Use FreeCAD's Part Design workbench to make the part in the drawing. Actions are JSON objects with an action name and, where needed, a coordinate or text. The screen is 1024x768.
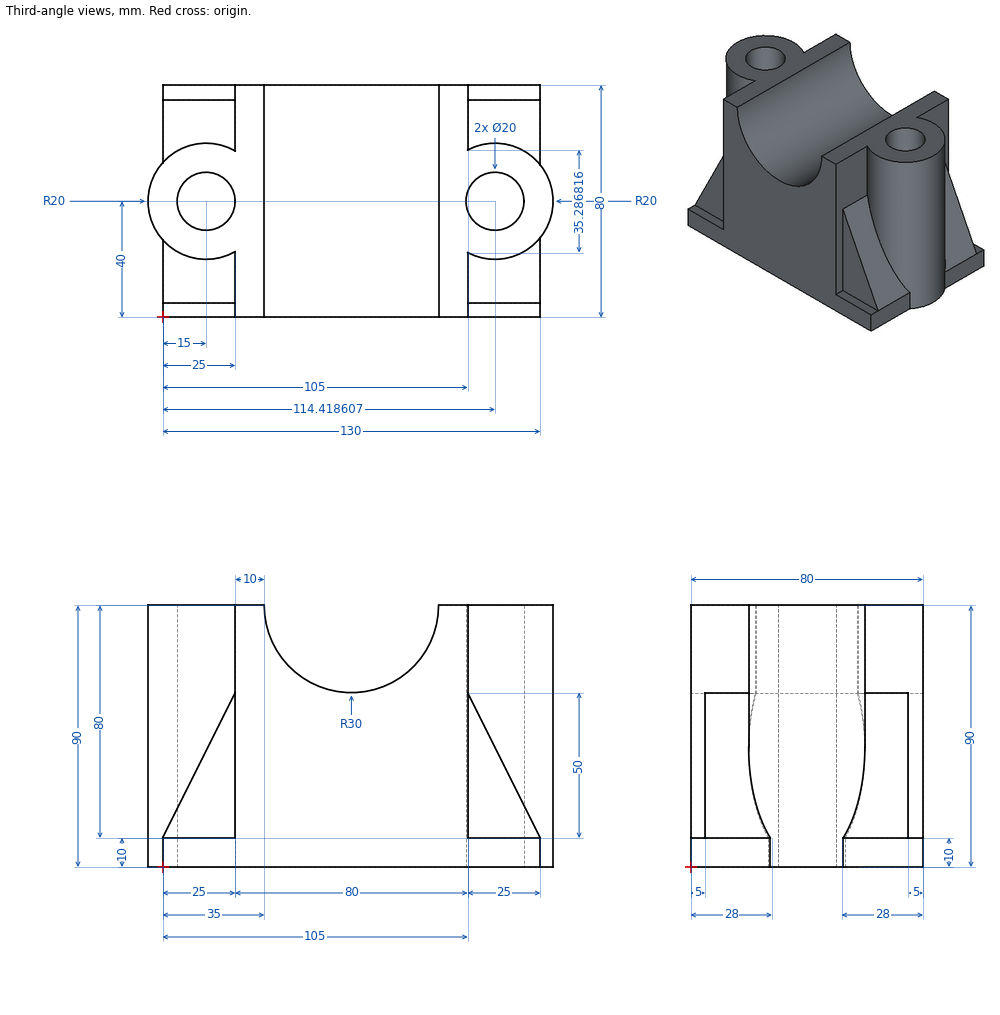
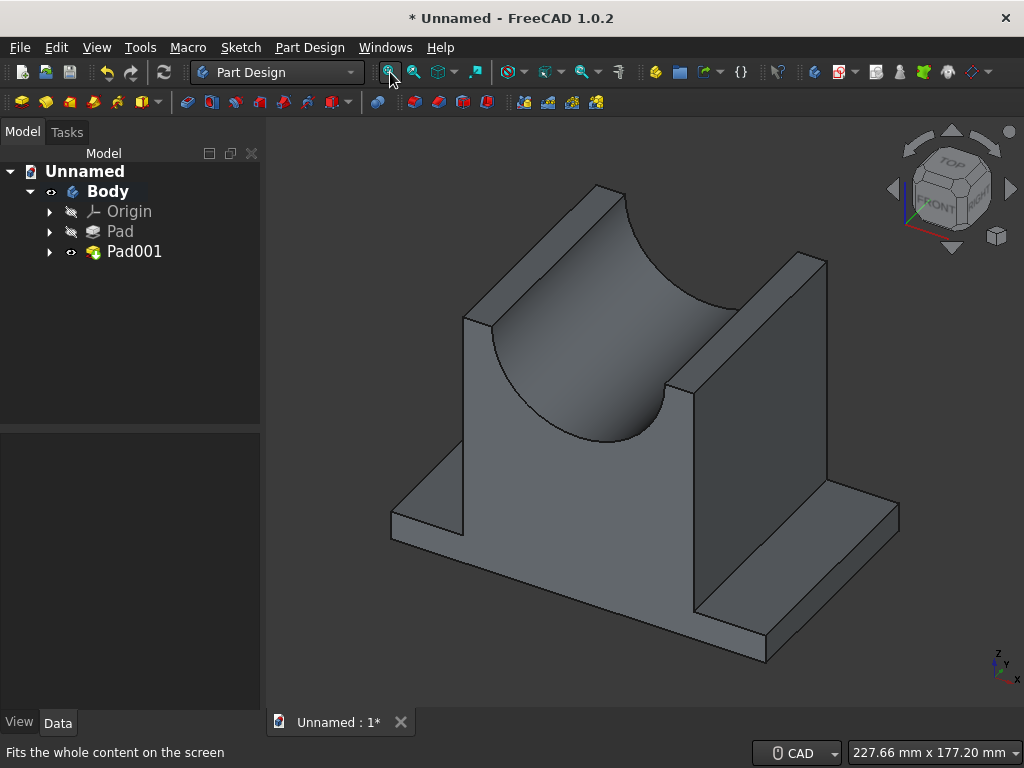
{"action": "left_click", "coordinate": [601, 198]}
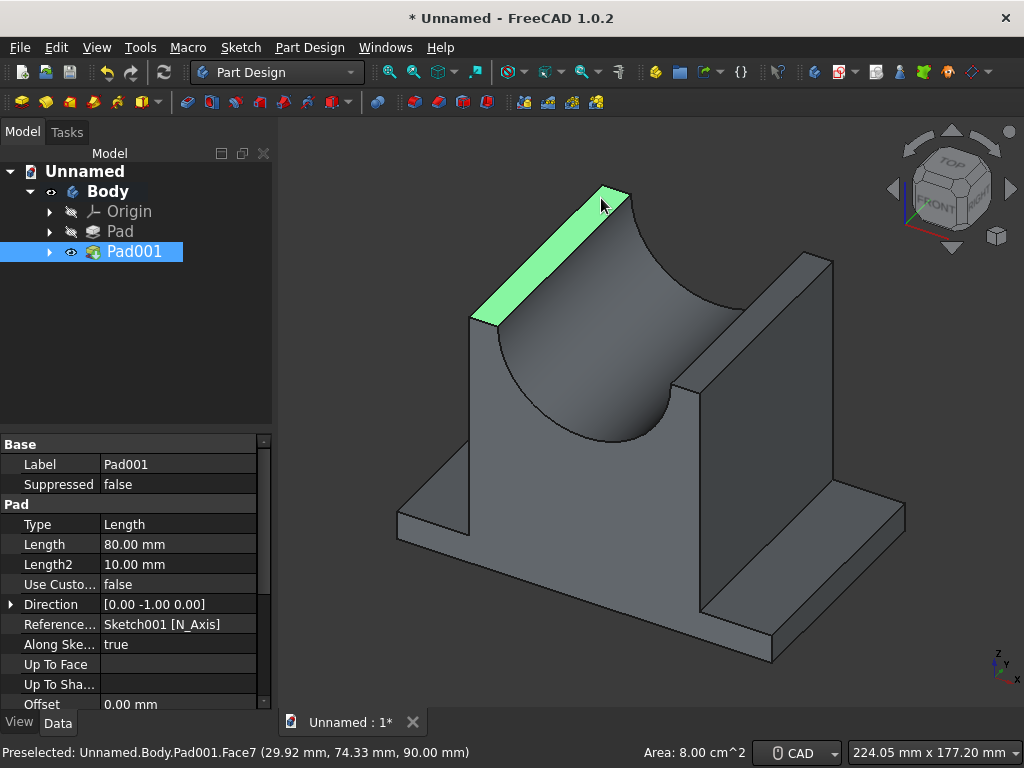
{"action": "left_click", "coordinate": [840, 72]}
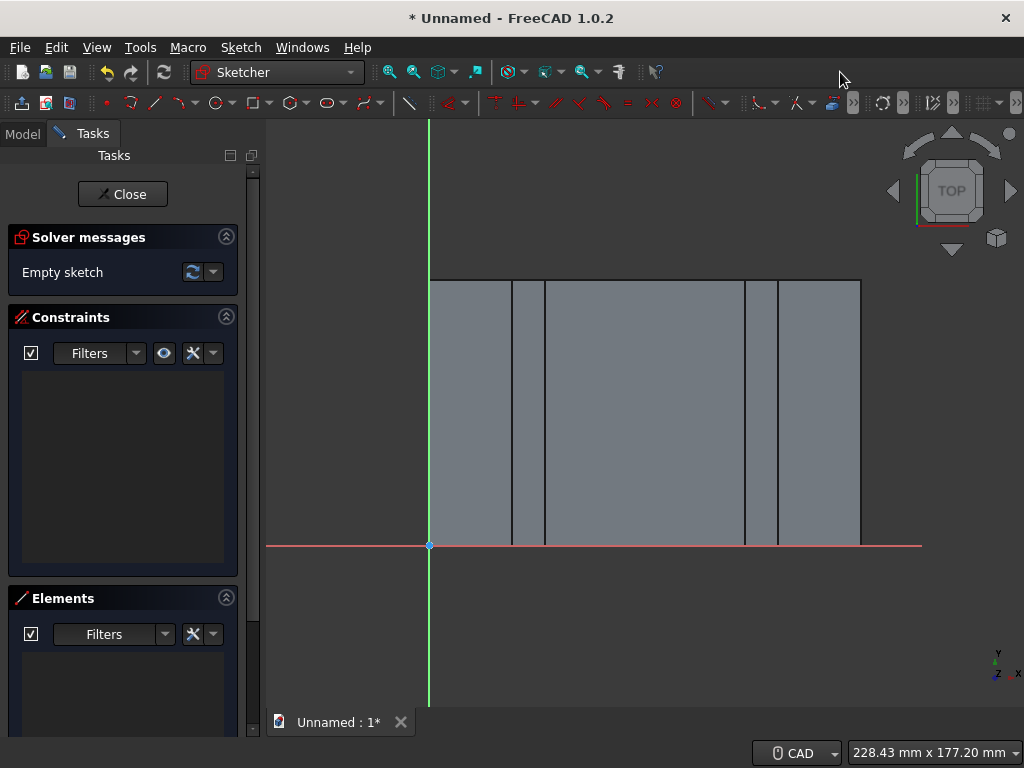
{"action": "scroll", "coordinate": [576, 413], "scroll_direction": "down", "scroll_amount": 5}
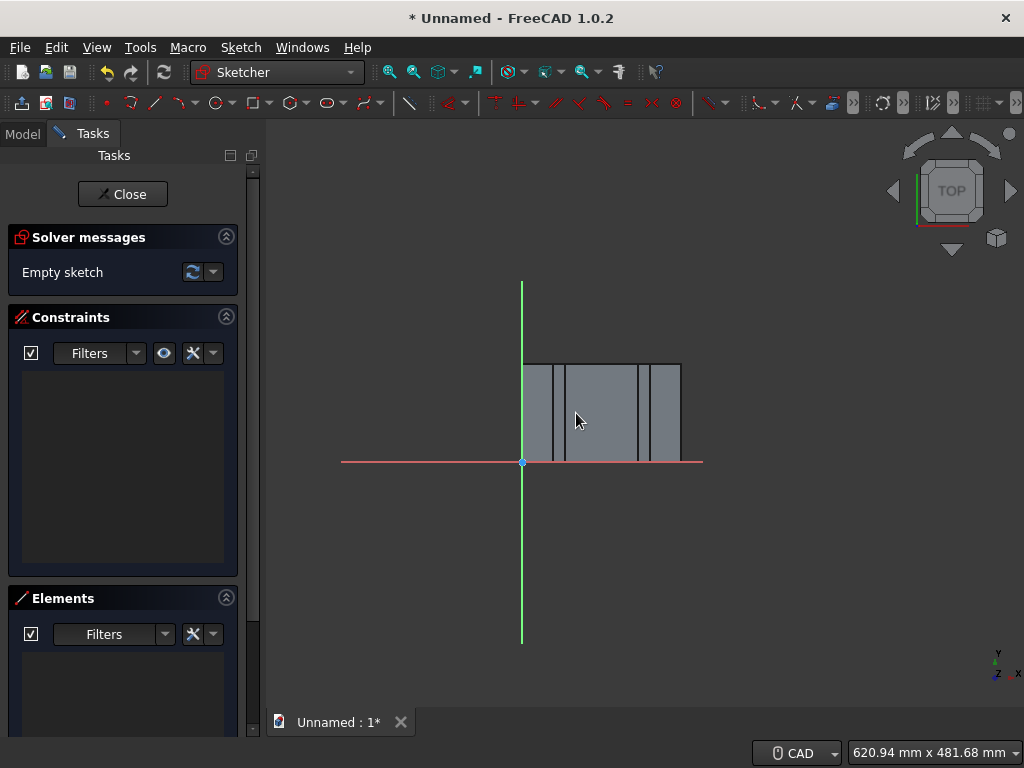
{"action": "scroll", "coordinate": [680, 413], "scroll_direction": "up", "scroll_amount": 11}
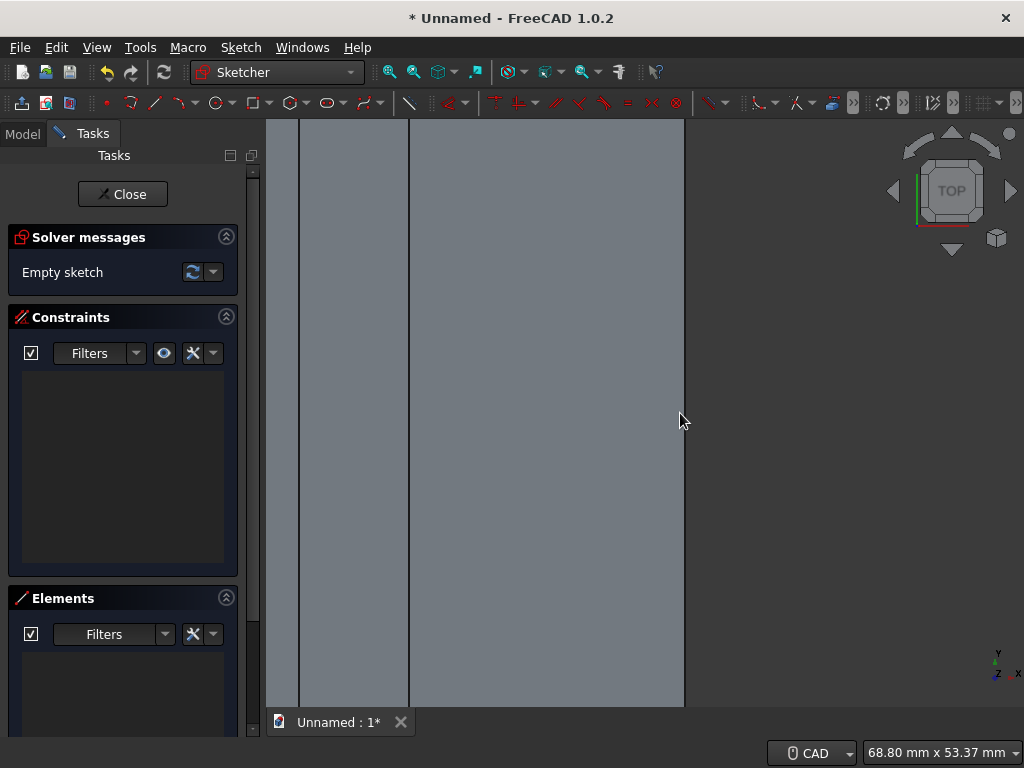
{"action": "left_click", "coordinate": [156, 104]}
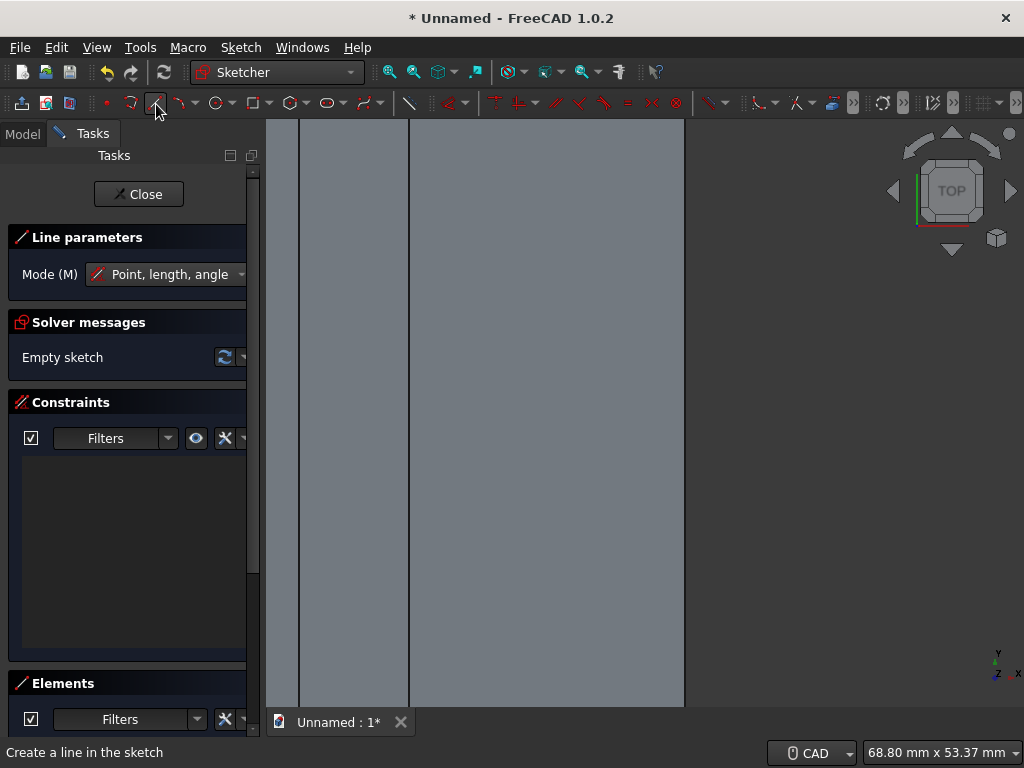
{"action": "left_click", "coordinate": [409, 217]}
{"action": "left_click", "coordinate": [409, 606]}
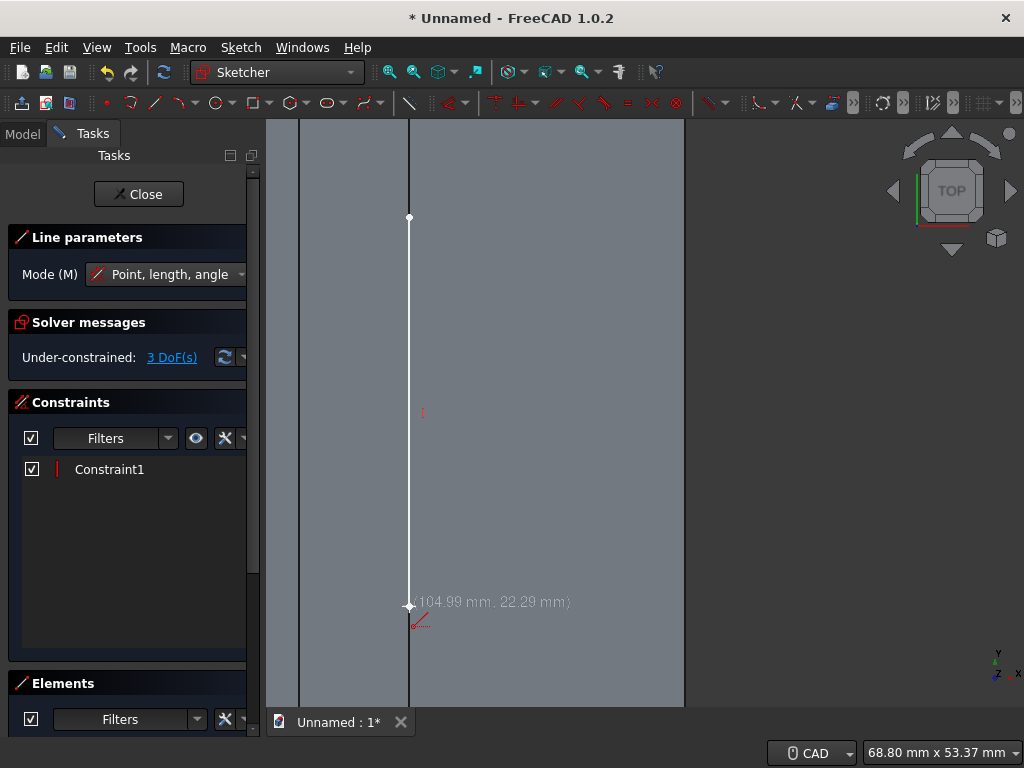
{"action": "left_click", "coordinate": [180, 104]}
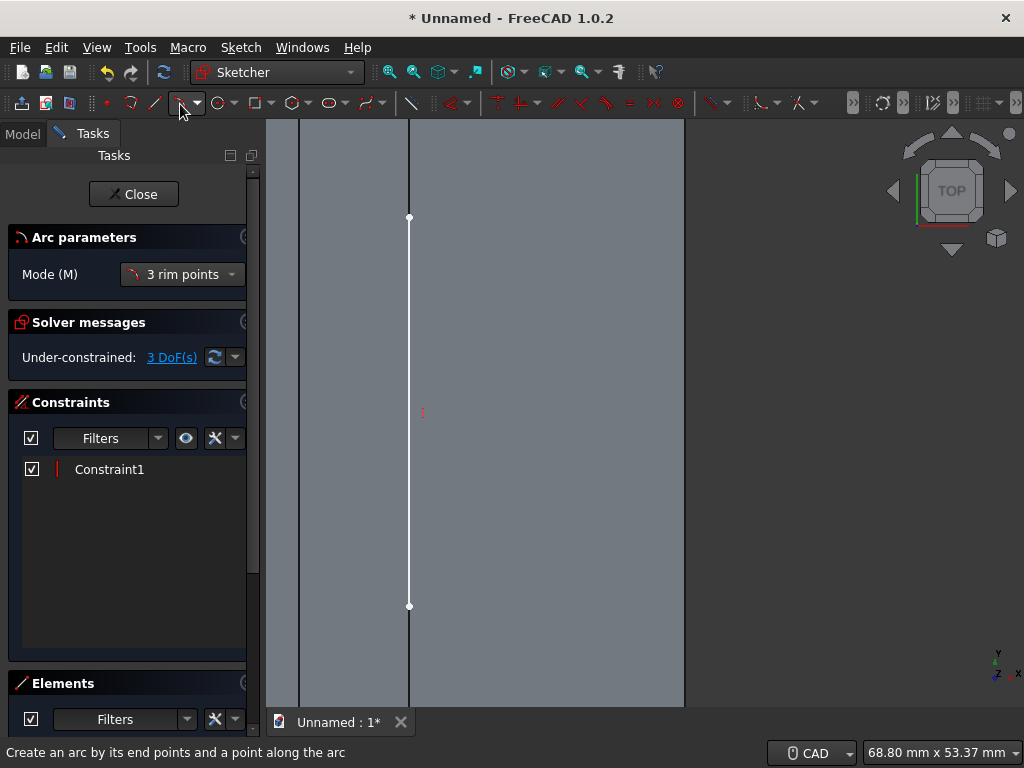
{"action": "left_click", "coordinate": [409, 607]}
{"action": "left_click", "coordinate": [409, 218]}
{"action": "left_click", "coordinate": [733, 412]}
{"action": "key", "text": "Escape"}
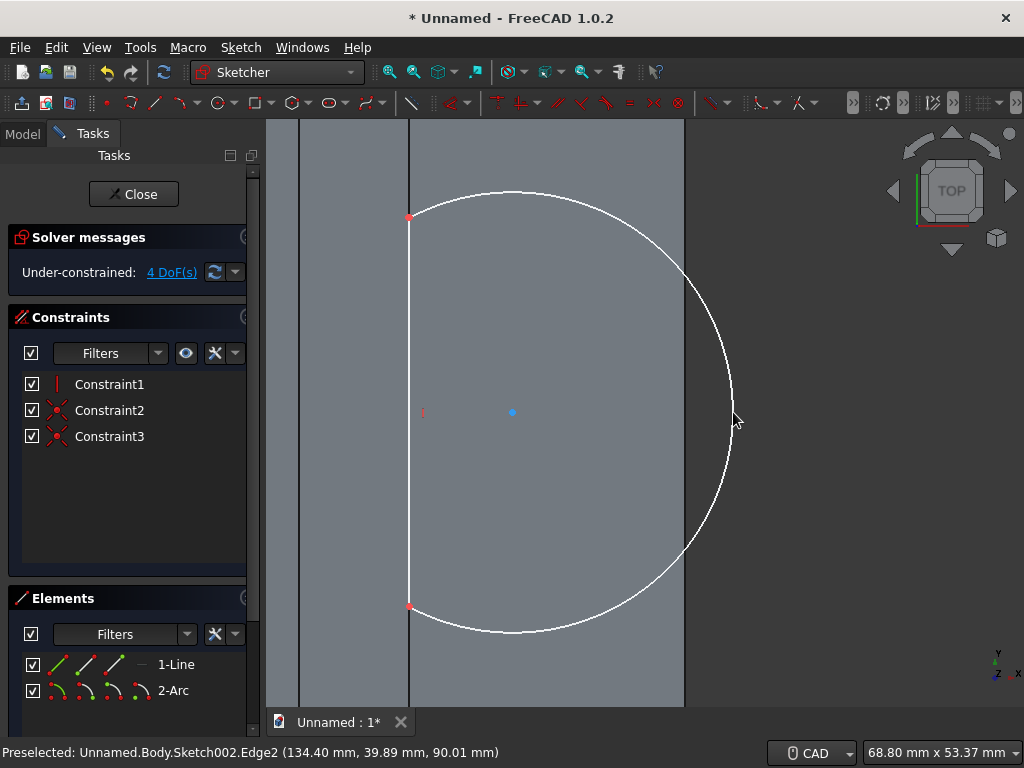
{"action": "left_click", "coordinate": [450, 104]}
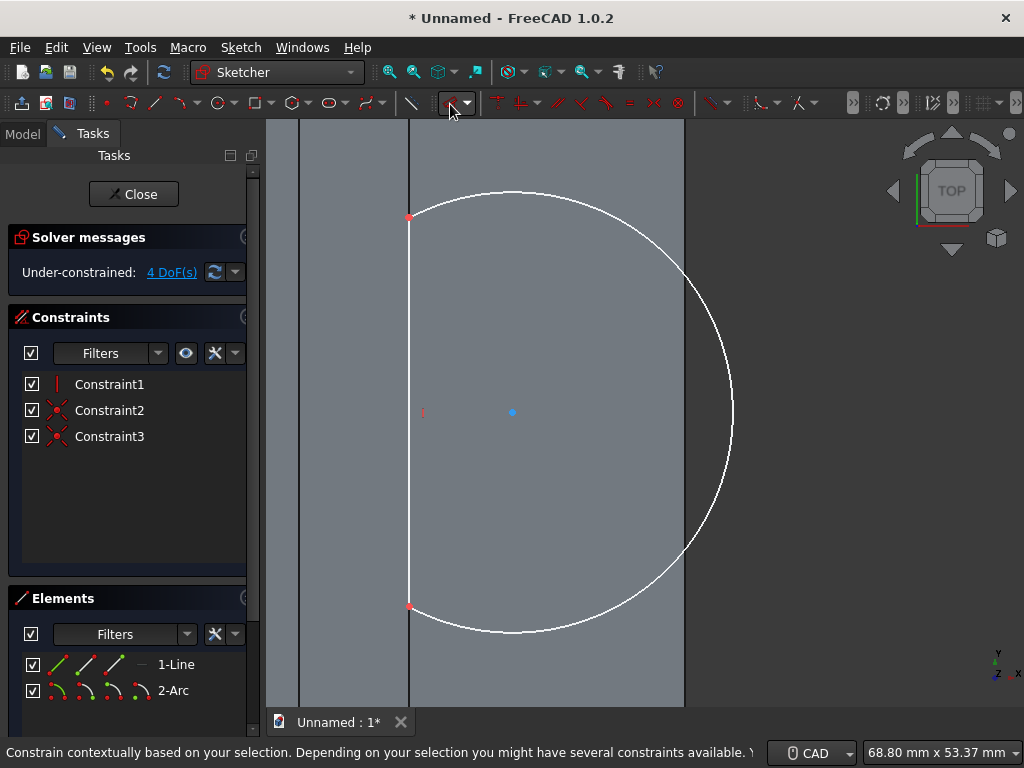
{"action": "left_click", "coordinate": [662, 574]}
{"action": "left_click", "coordinate": [684, 597]}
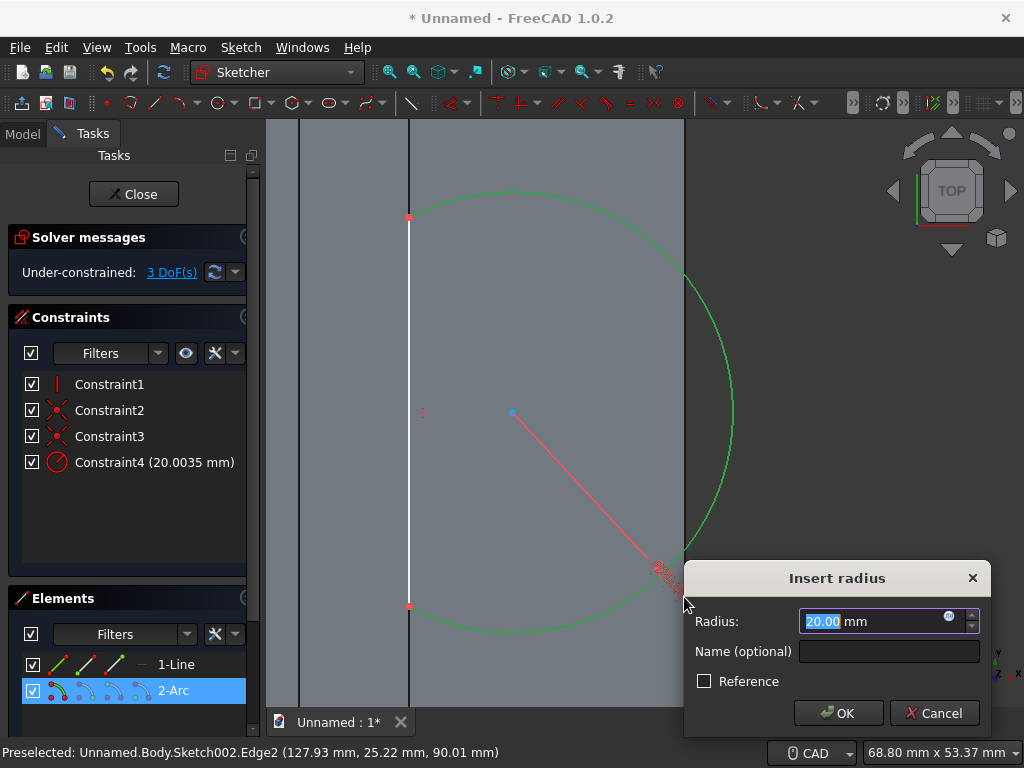
{"action": "type", "text": "20"}
{"action": "key", "text": "Return"}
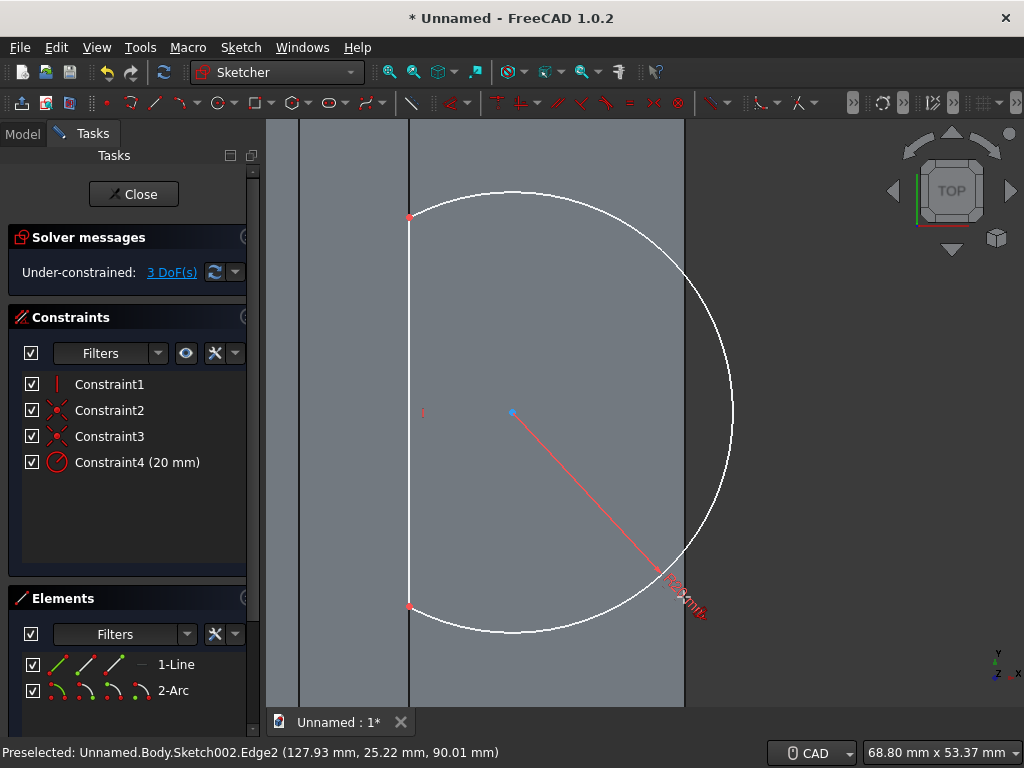
{"action": "left_click", "coordinate": [513, 413]}
{"action": "left_click", "coordinate": [547, 546]}